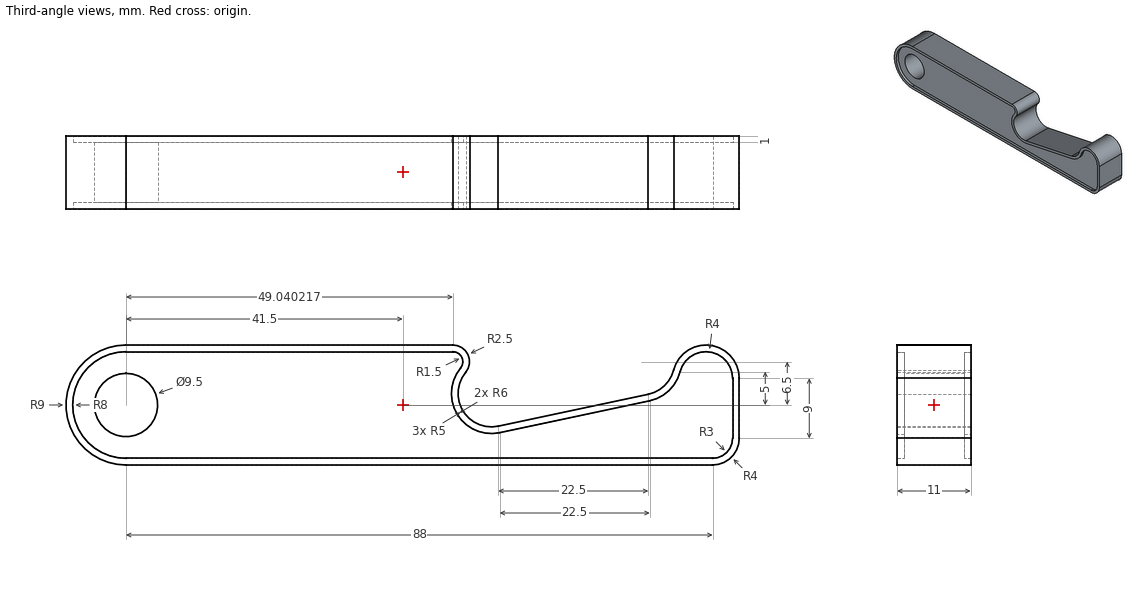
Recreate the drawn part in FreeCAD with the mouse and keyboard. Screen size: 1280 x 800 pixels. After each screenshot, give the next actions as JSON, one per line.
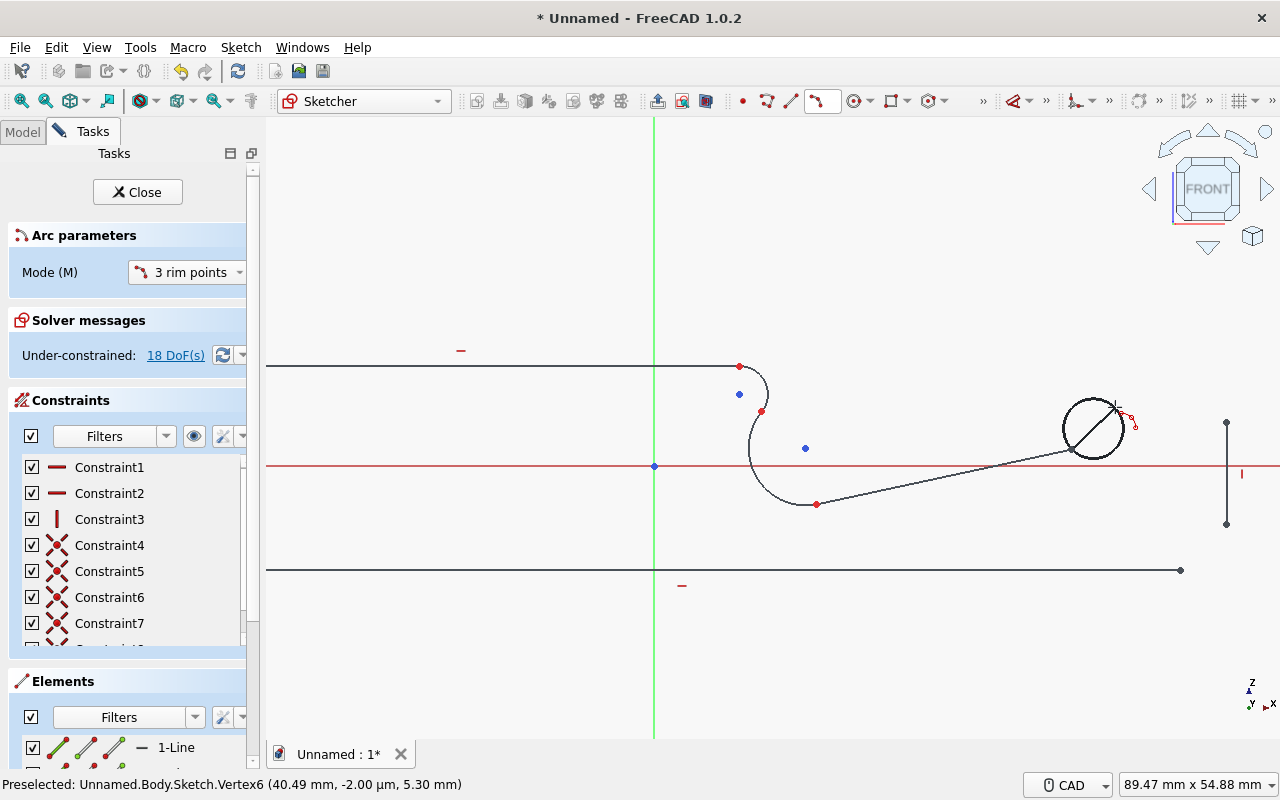
{"action": "scroll", "coordinate": [1099, 434], "scroll_direction": "up", "scroll_amount": 4}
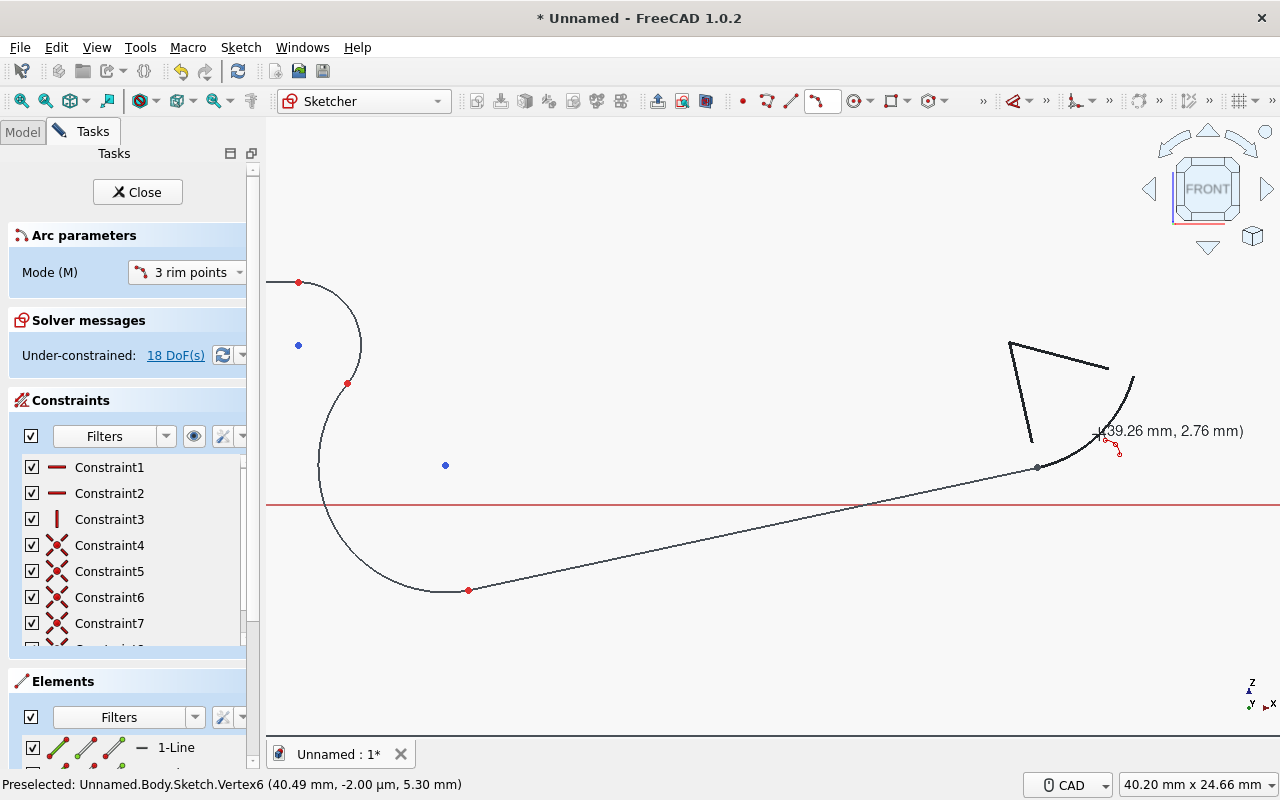
{"action": "left_click", "coordinate": [1098, 432]}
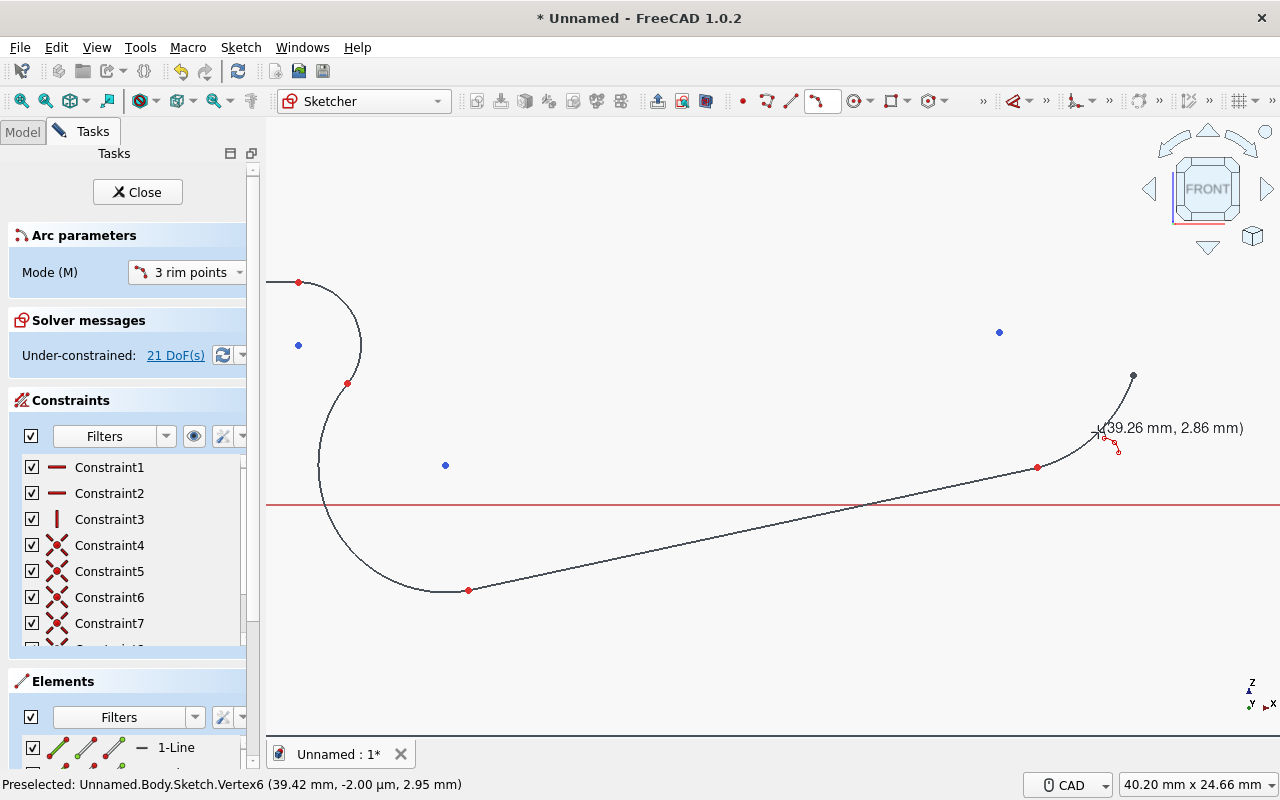
{"action": "scroll", "coordinate": [900, 403], "scroll_direction": "down", "scroll_amount": 7}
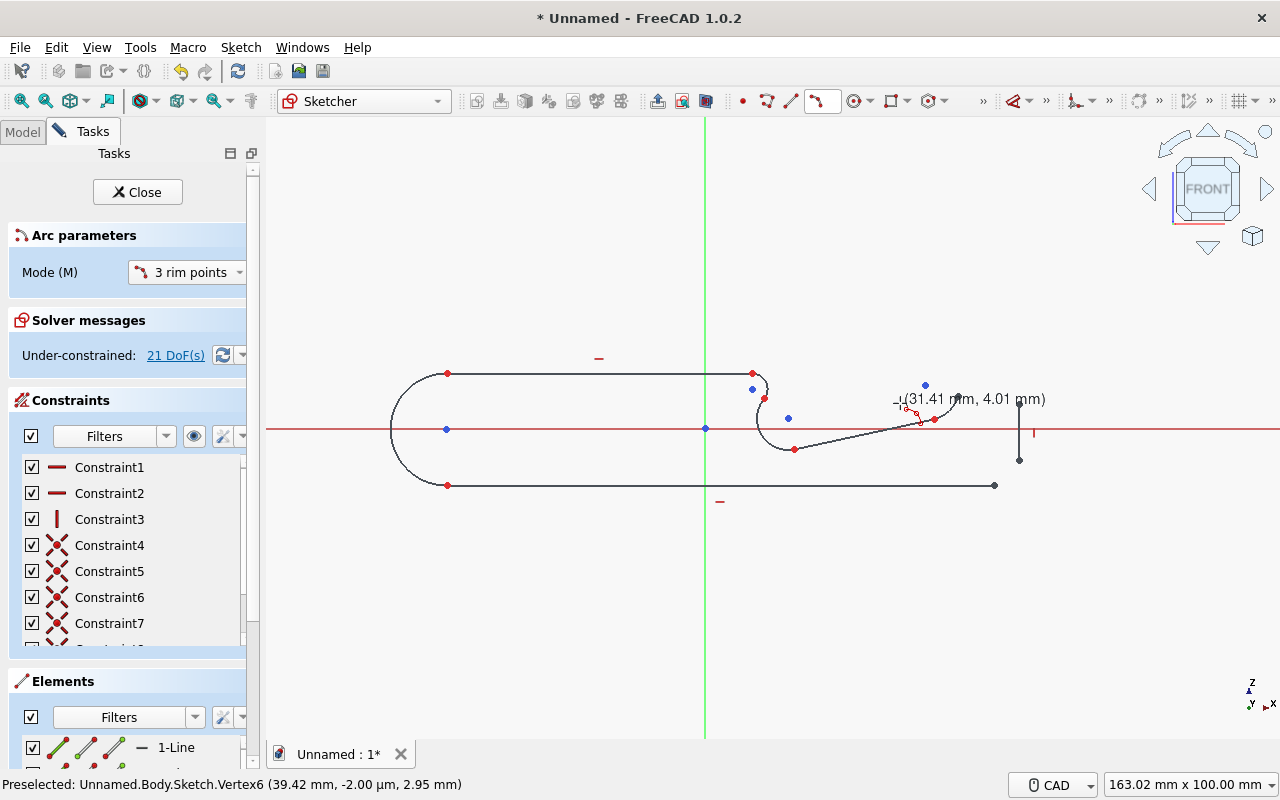
{"action": "left_click", "coordinate": [958, 397]}
{"action": "left_click", "coordinate": [1019, 405]}
{"action": "left_click", "coordinate": [992, 373]}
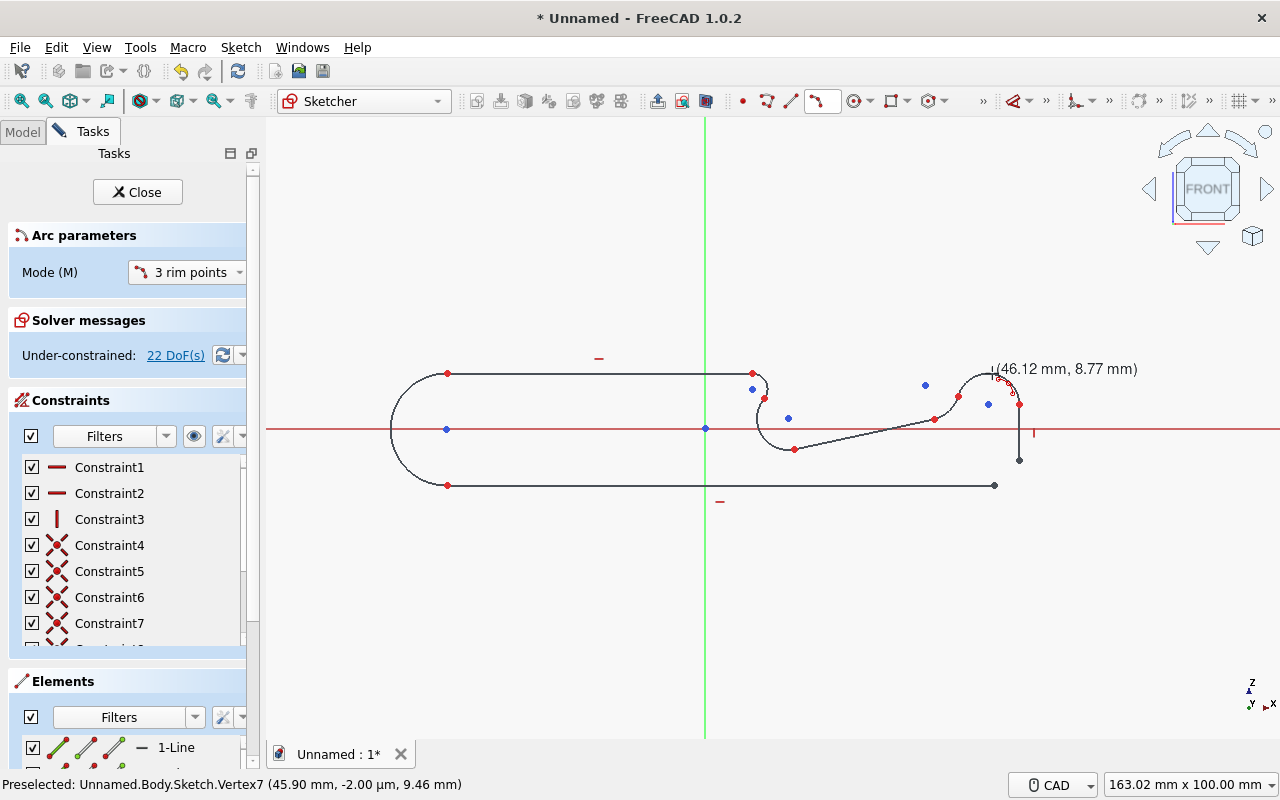
{"action": "left_click", "coordinate": [1019, 461]}
{"action": "left_click", "coordinate": [994, 486]}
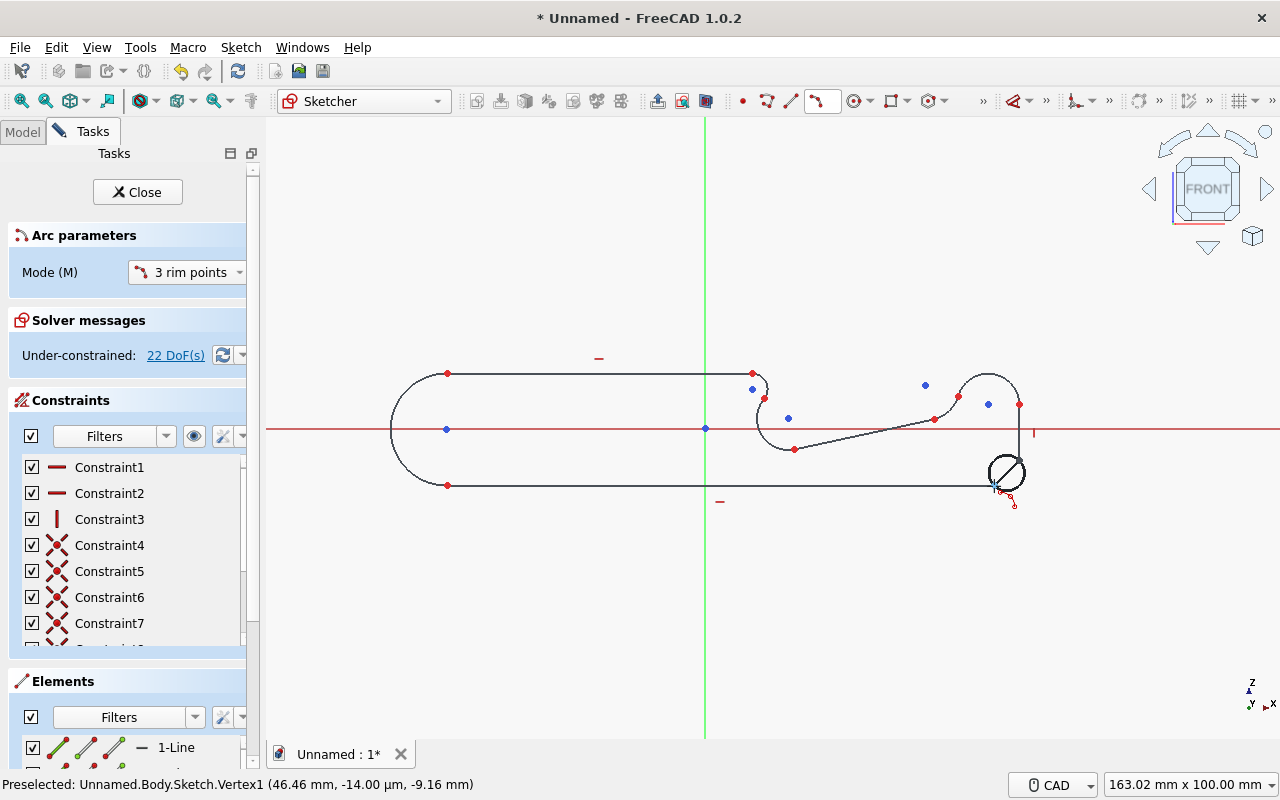
{"action": "scroll", "coordinate": [1012, 477], "scroll_direction": "up", "scroll_amount": 4}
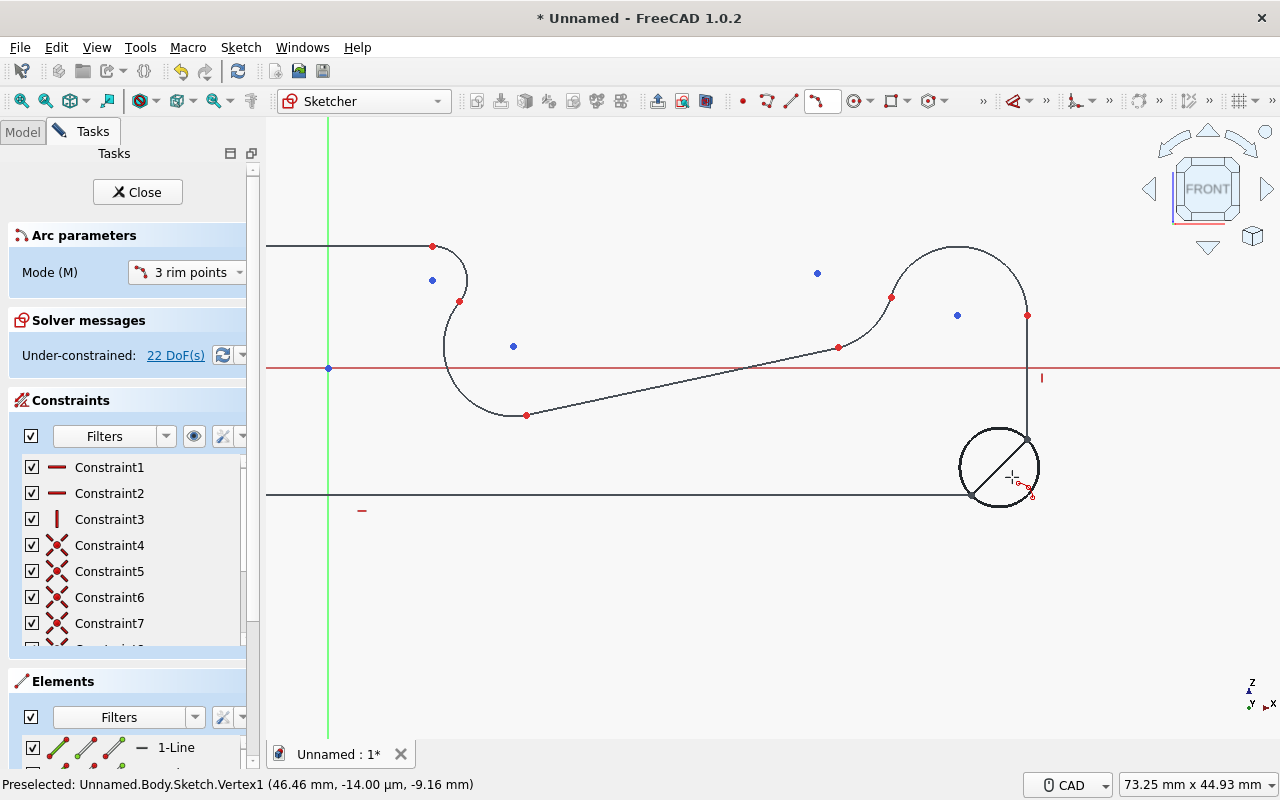
{"action": "left_click", "coordinate": [1011, 477]}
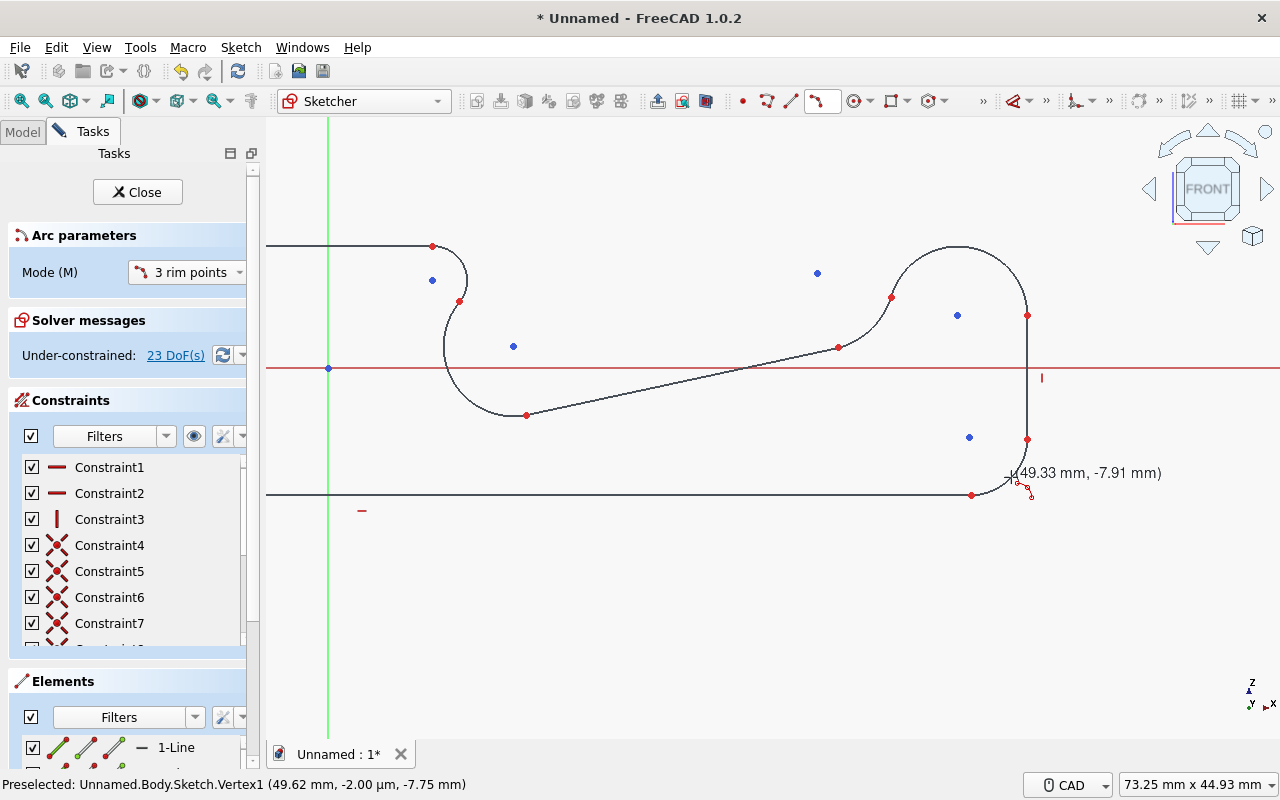
{"action": "key", "text": "g c"}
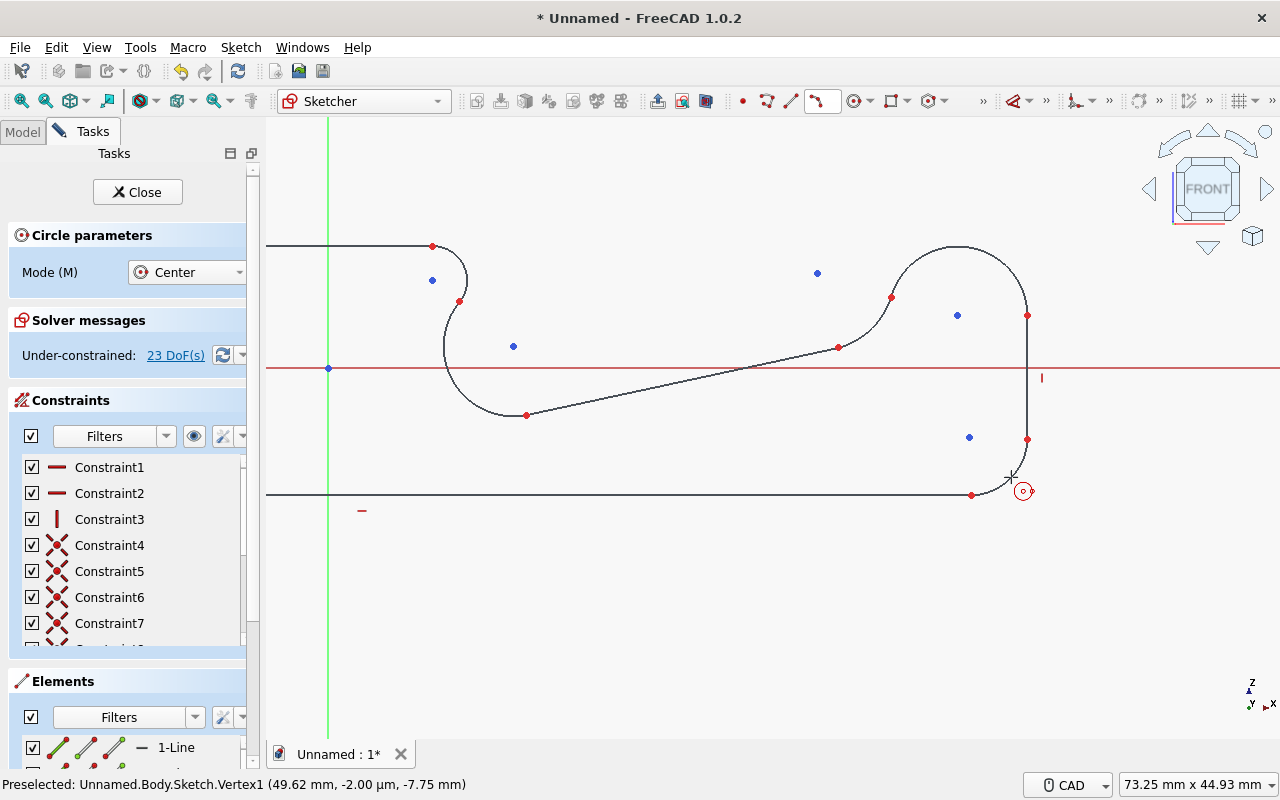
{"action": "scroll", "coordinate": [1012, 477], "scroll_direction": "down", "scroll_amount": 4}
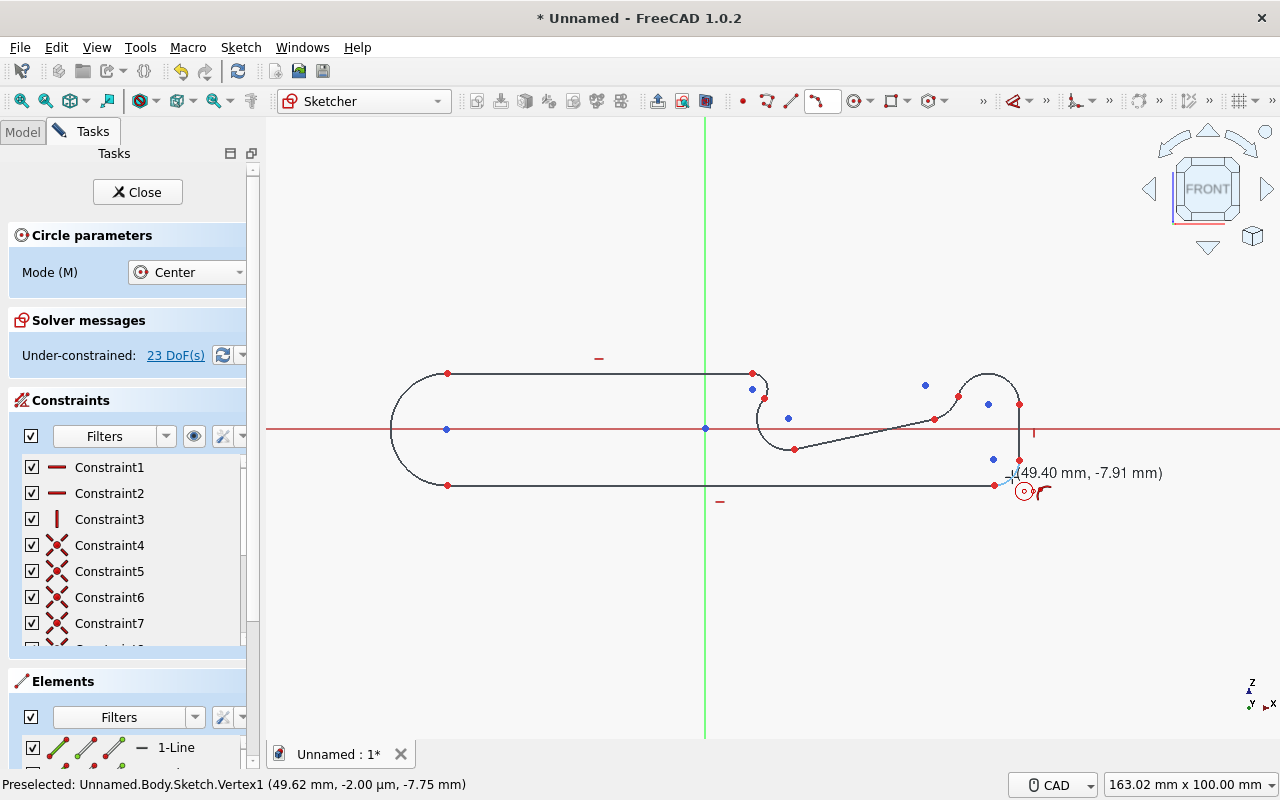
{"action": "left_click", "coordinate": [447, 429]}
{"action": "mouse_move", "coordinate": [468, 408]}